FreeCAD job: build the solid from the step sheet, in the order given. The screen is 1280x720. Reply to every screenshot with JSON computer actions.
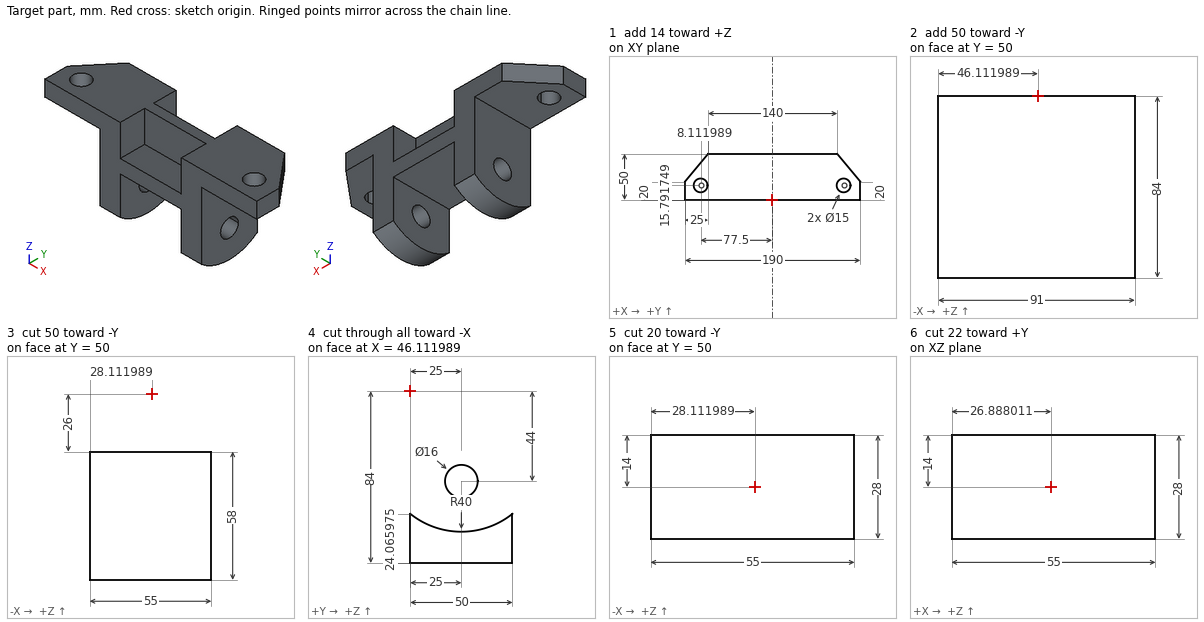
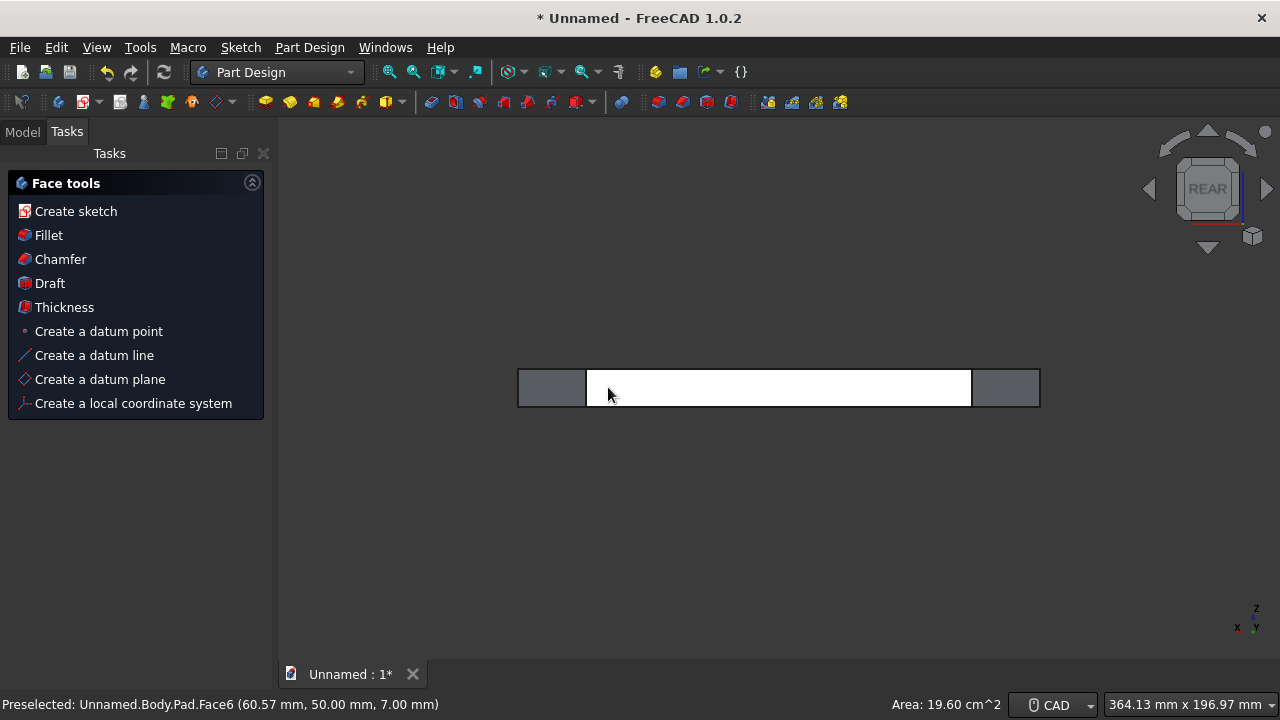
{"action": "left_click", "coordinate": [84, 102]}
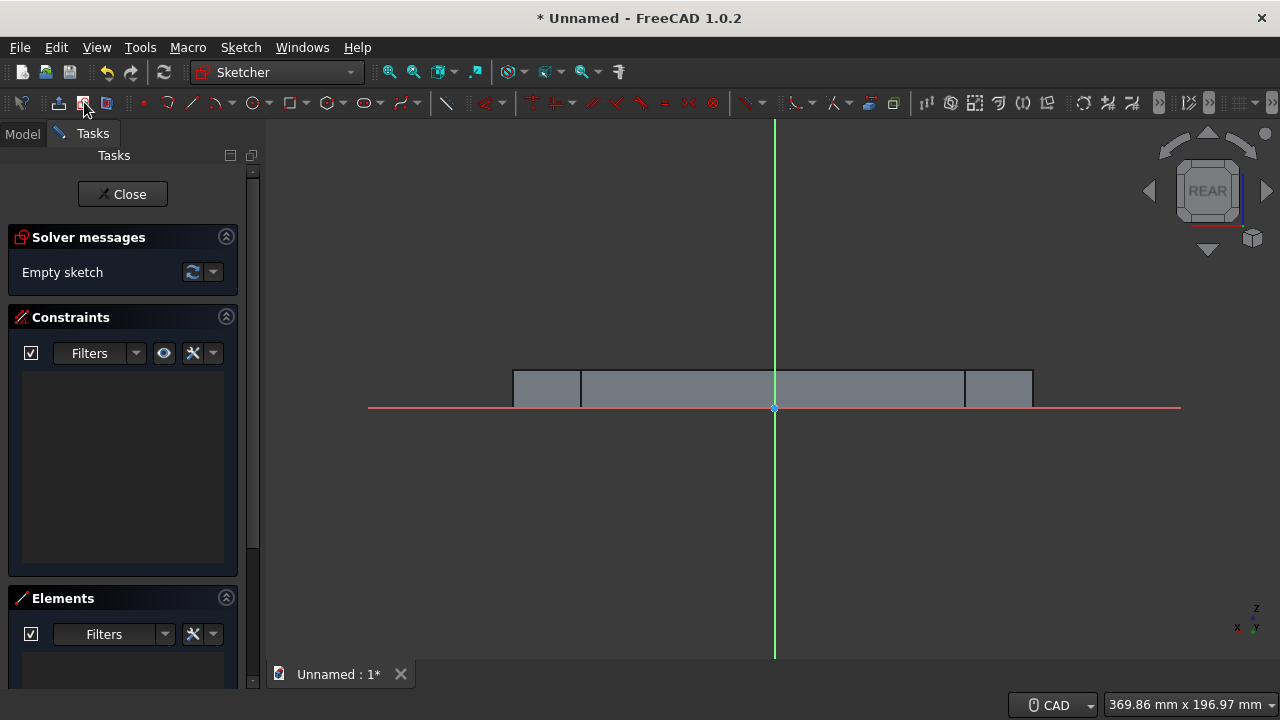
{"action": "scroll", "coordinate": [395, 147], "scroll_direction": "down", "scroll_amount": 1}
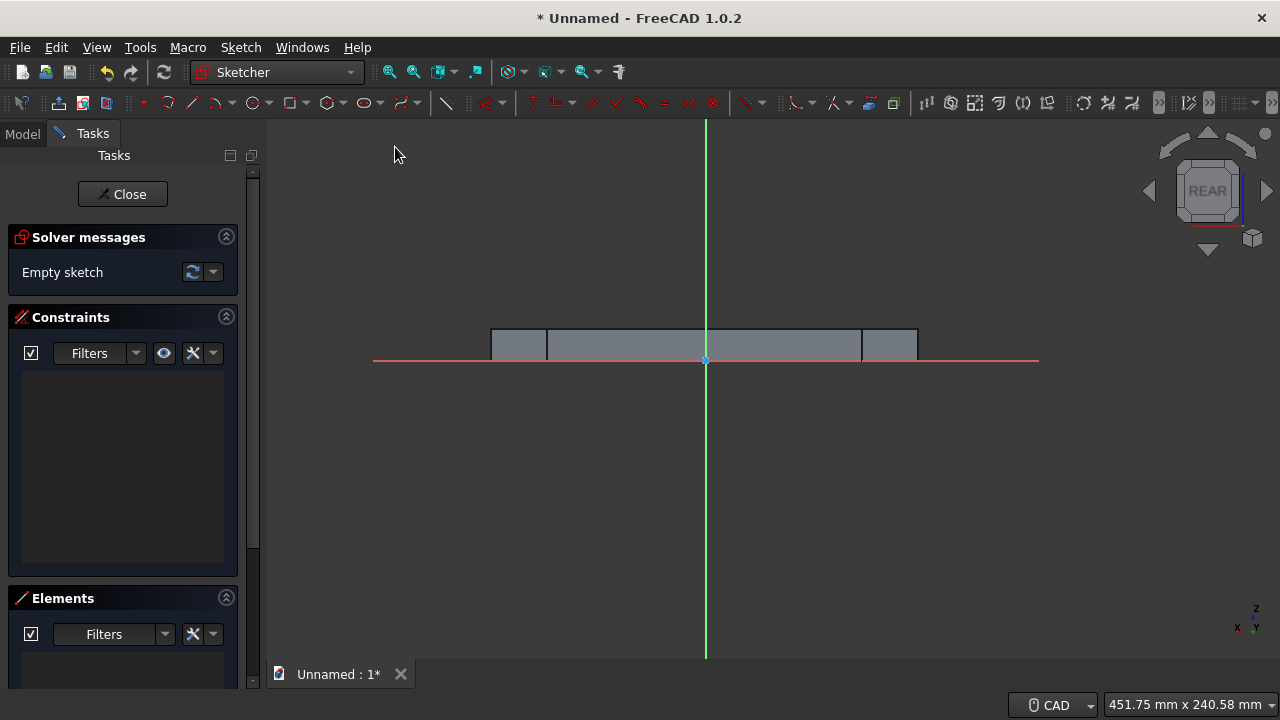
{"action": "scroll", "coordinate": [705, 536], "scroll_direction": "up", "scroll_amount": 3}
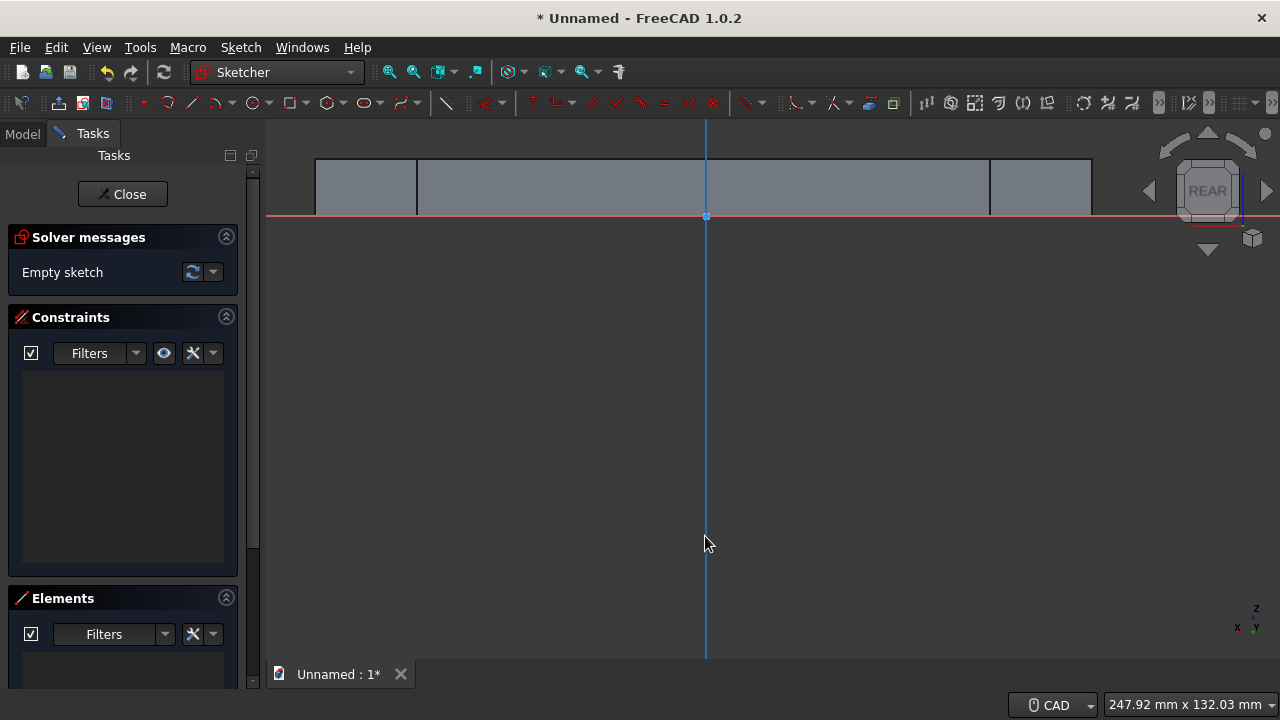
{"action": "left_click", "coordinate": [290, 104]}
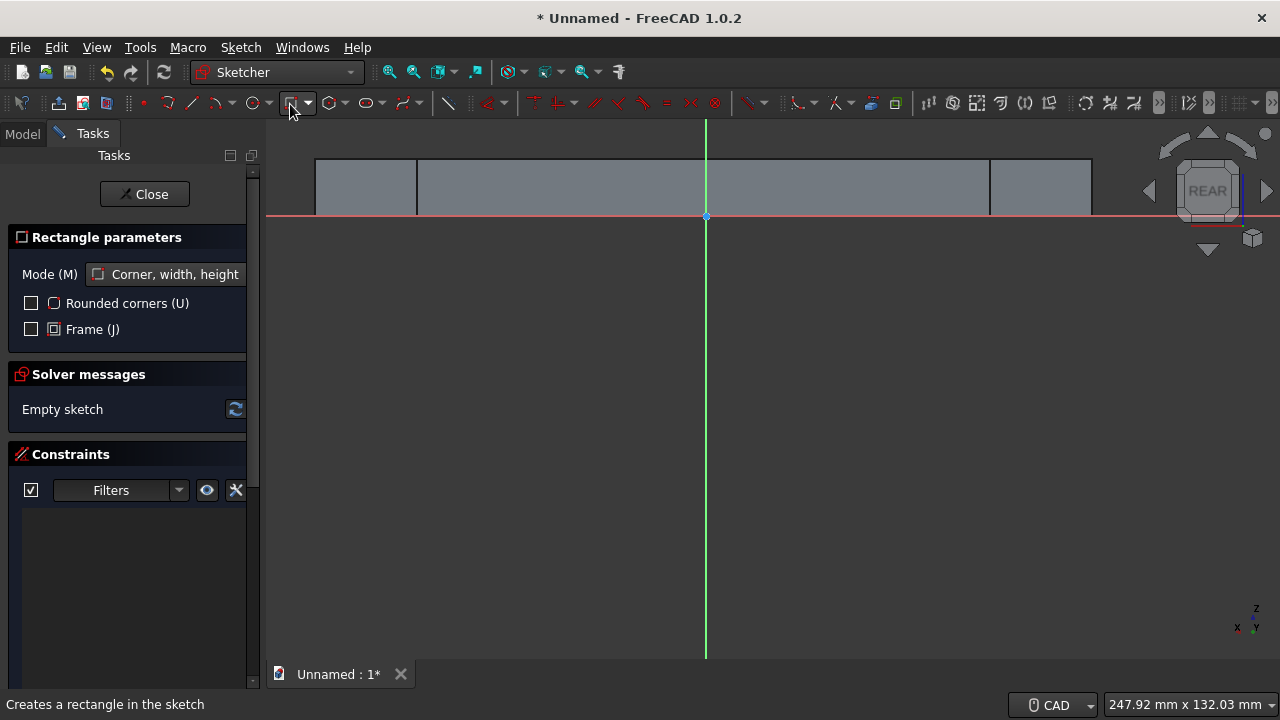
{"action": "left_click", "coordinate": [518, 216]}
{"action": "mouse_move", "coordinate": [890, 560]}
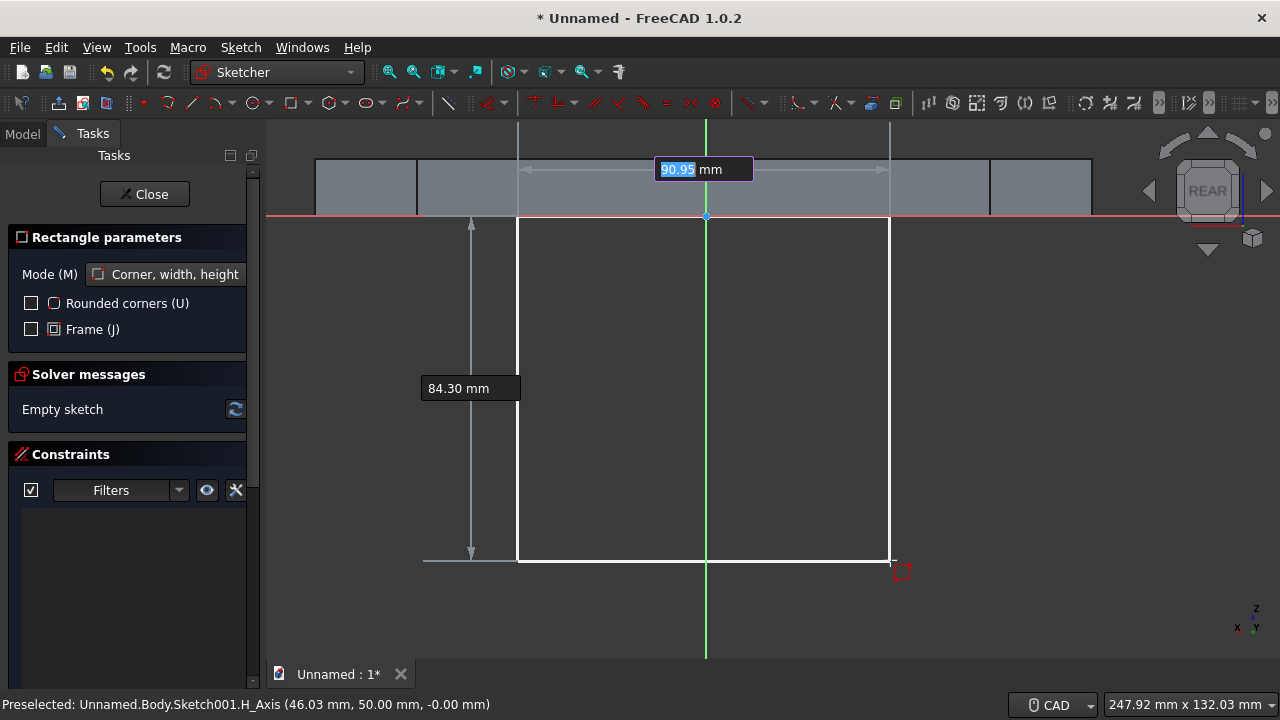
{"action": "type", "text": "91"}
{"action": "key", "text": "Tab"}
{"action": "type", "text": "84"}
{"action": "key", "text": "Return"}
{"action": "key", "text": "Escape"}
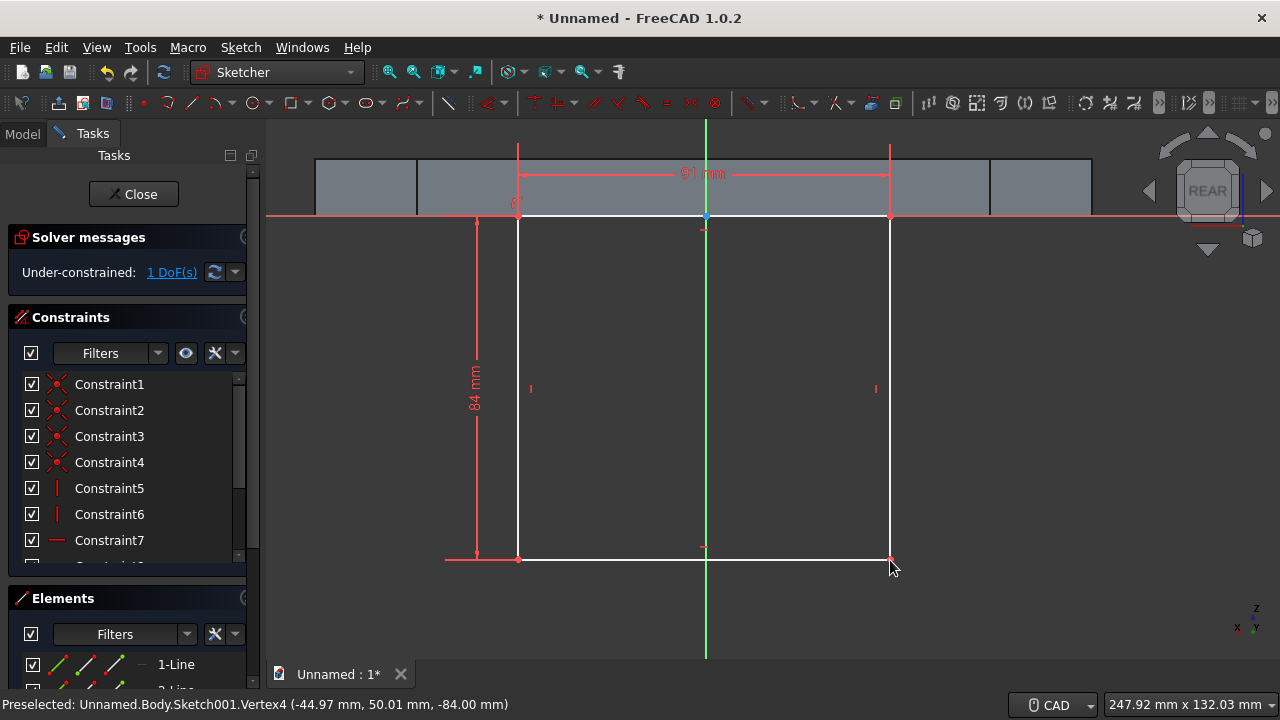
{"action": "left_click", "coordinate": [488, 104]}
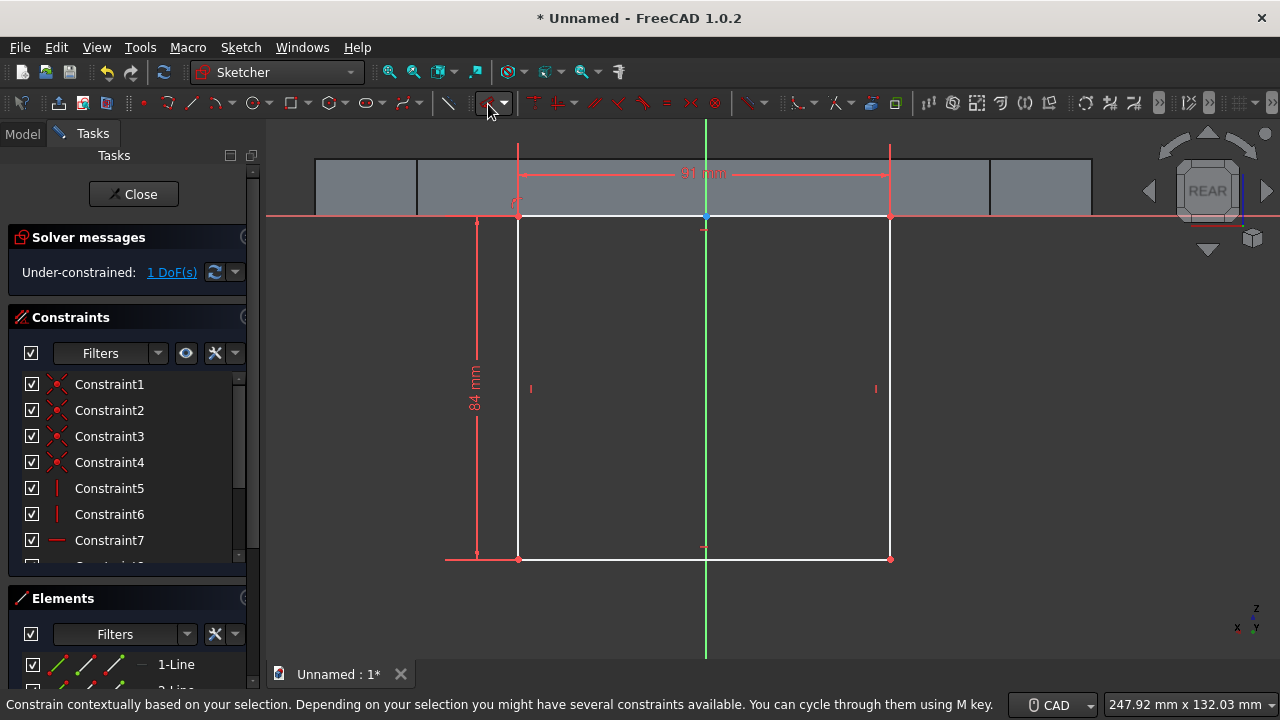
{"action": "left_click", "coordinate": [518, 216]}
{"action": "left_click", "coordinate": [612, 182]}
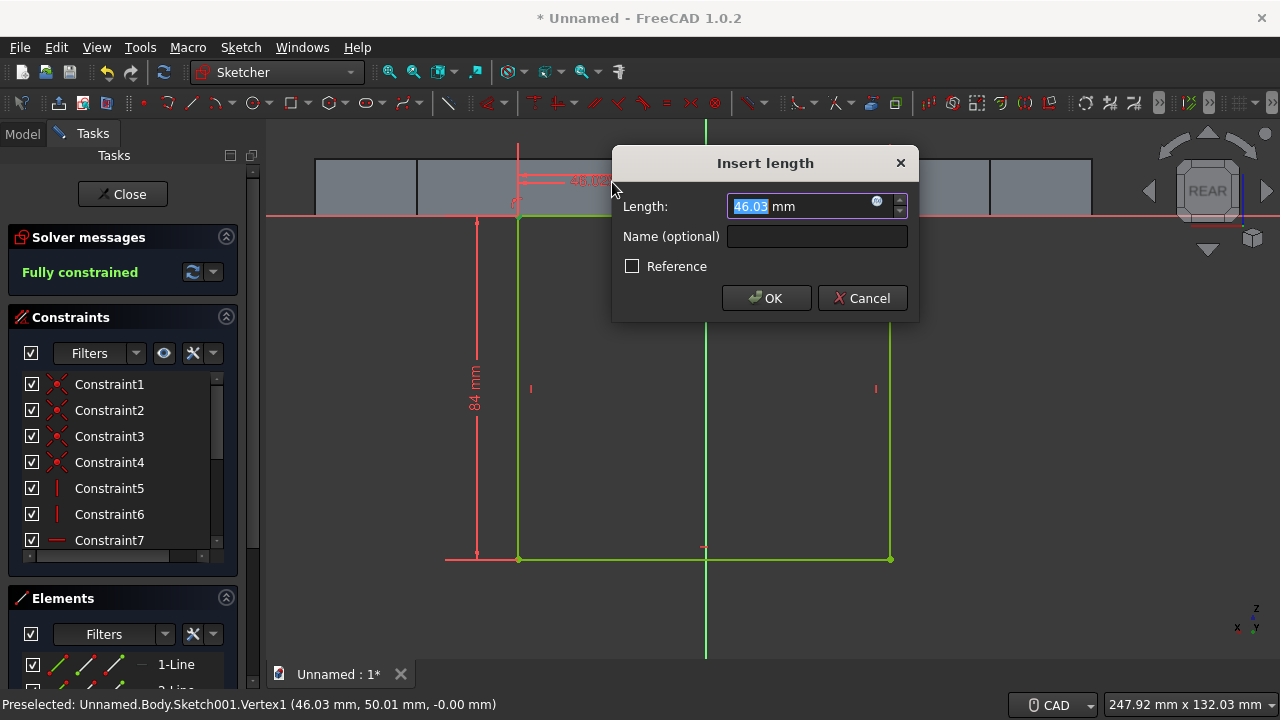
{"action": "type", "text": "46.111989"}
{"action": "key", "text": "Return"}
{"action": "key", "text": "Escape"}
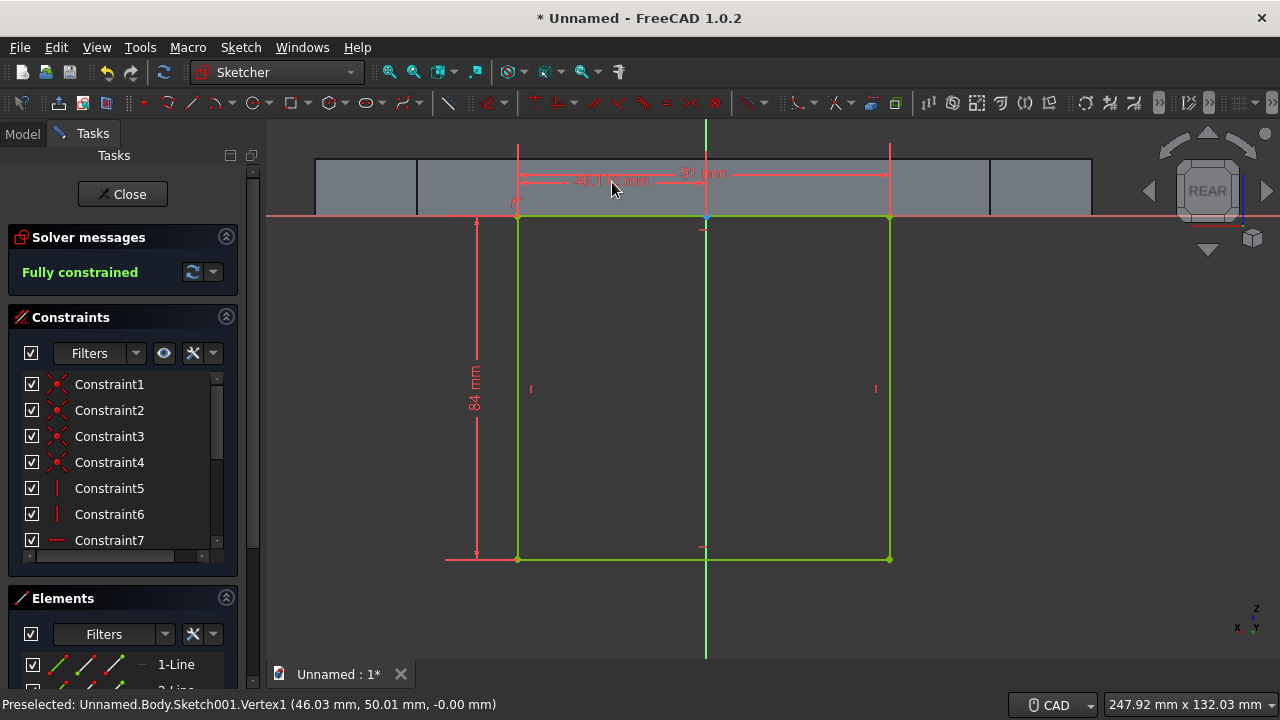
{"action": "left_click", "coordinate": [123, 194]}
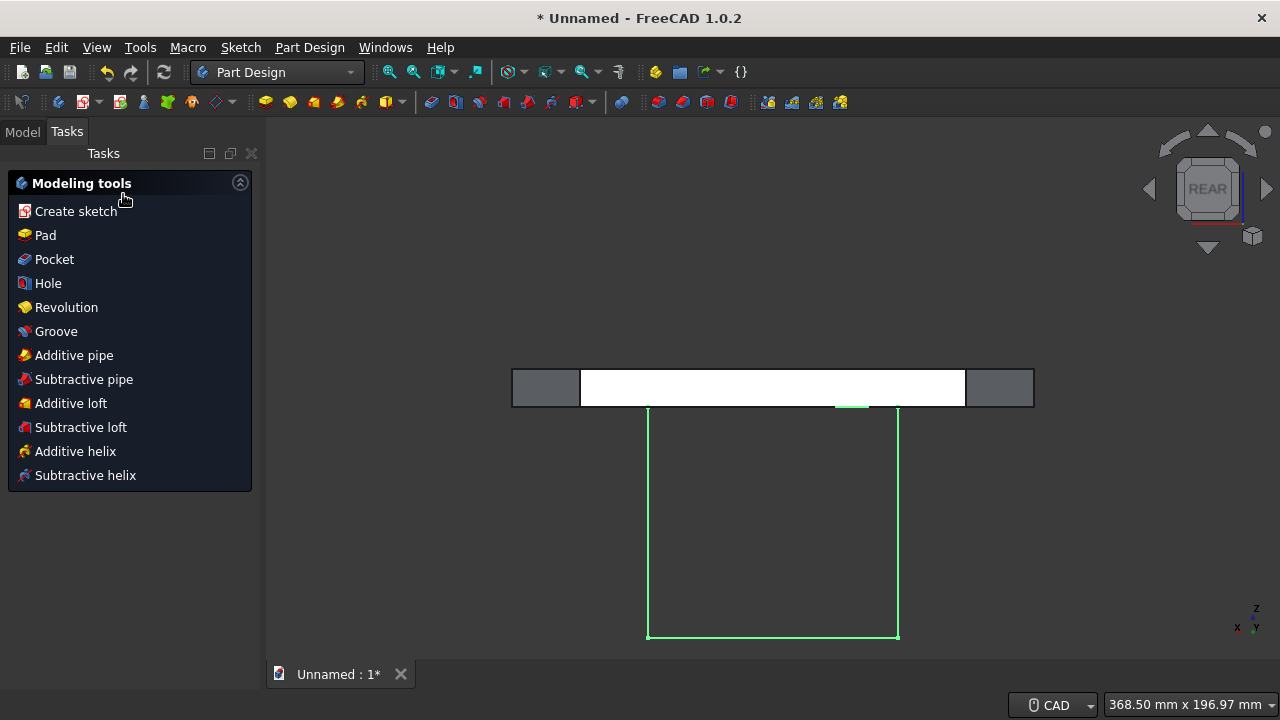
{"action": "left_click", "coordinate": [266, 102]}